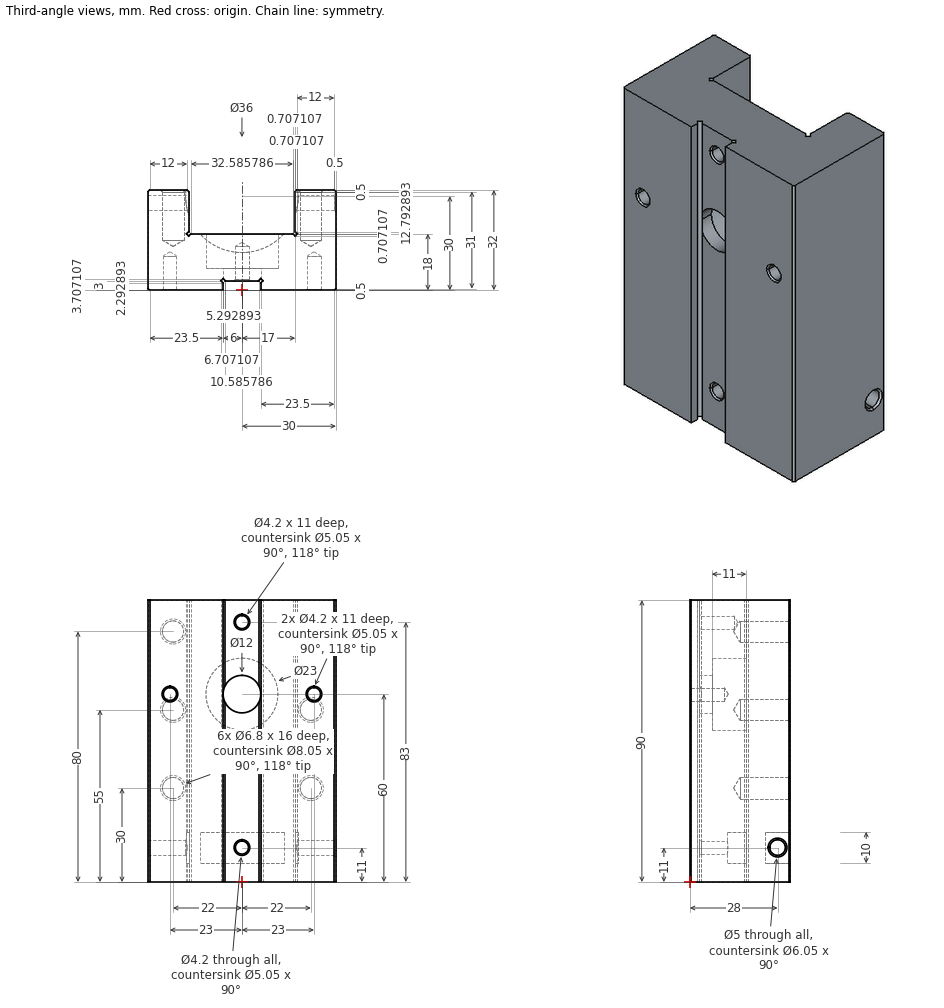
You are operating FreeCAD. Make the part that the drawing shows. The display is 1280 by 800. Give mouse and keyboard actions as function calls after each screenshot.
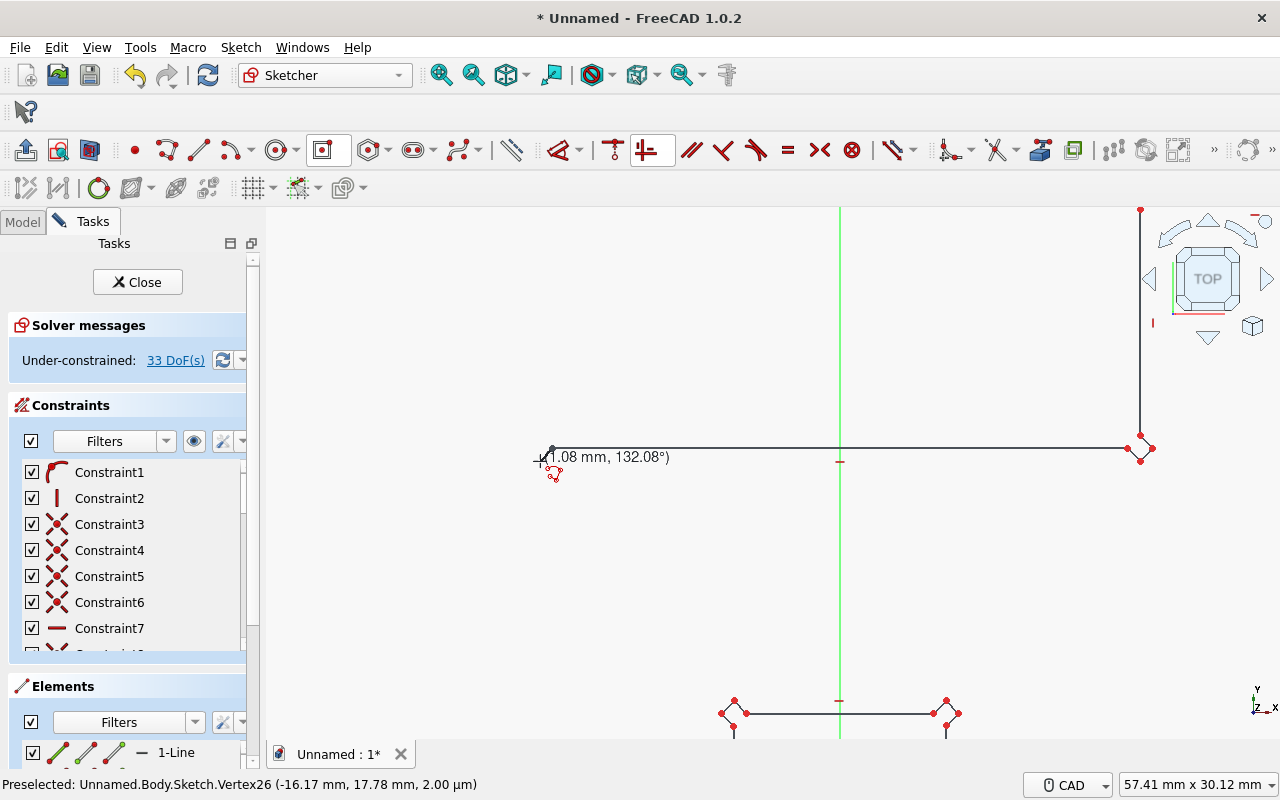
click(540, 460)
click(527, 448)
click(540, 435)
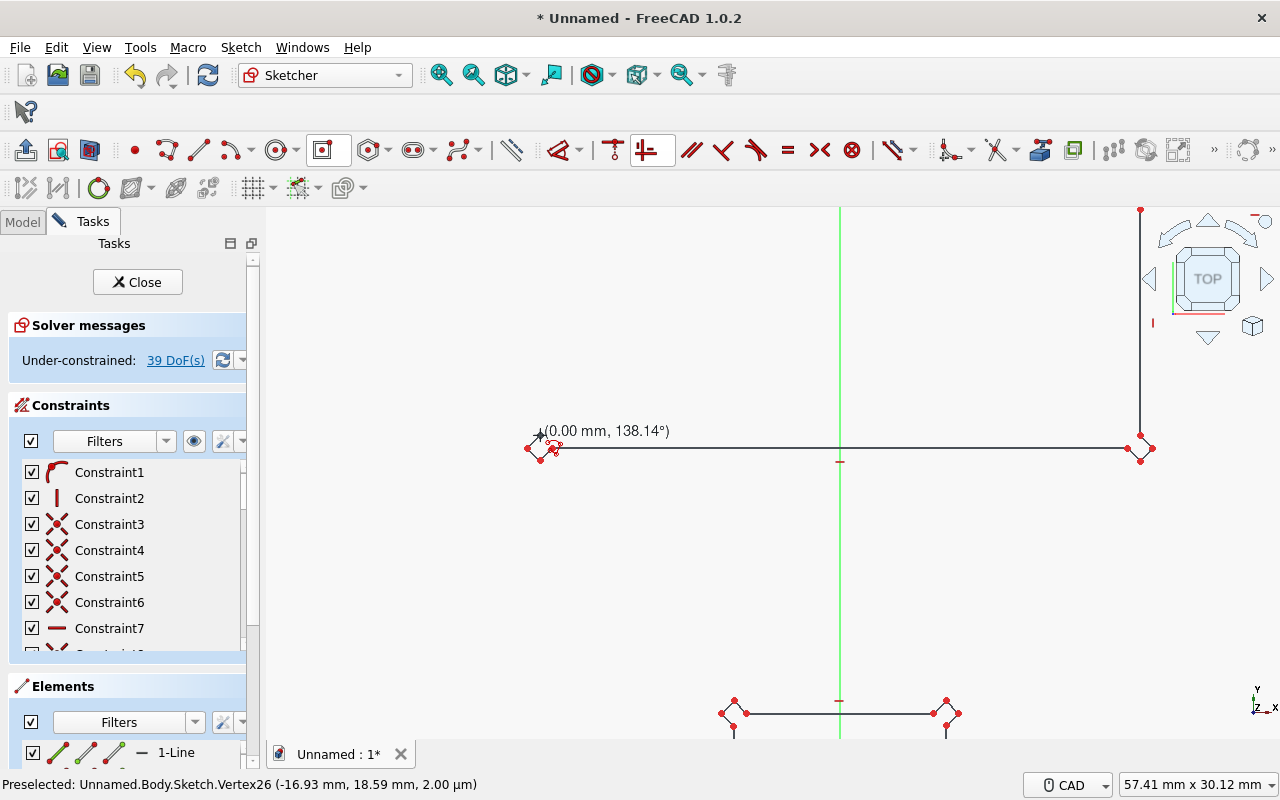
scroll(540, 461, down, 3)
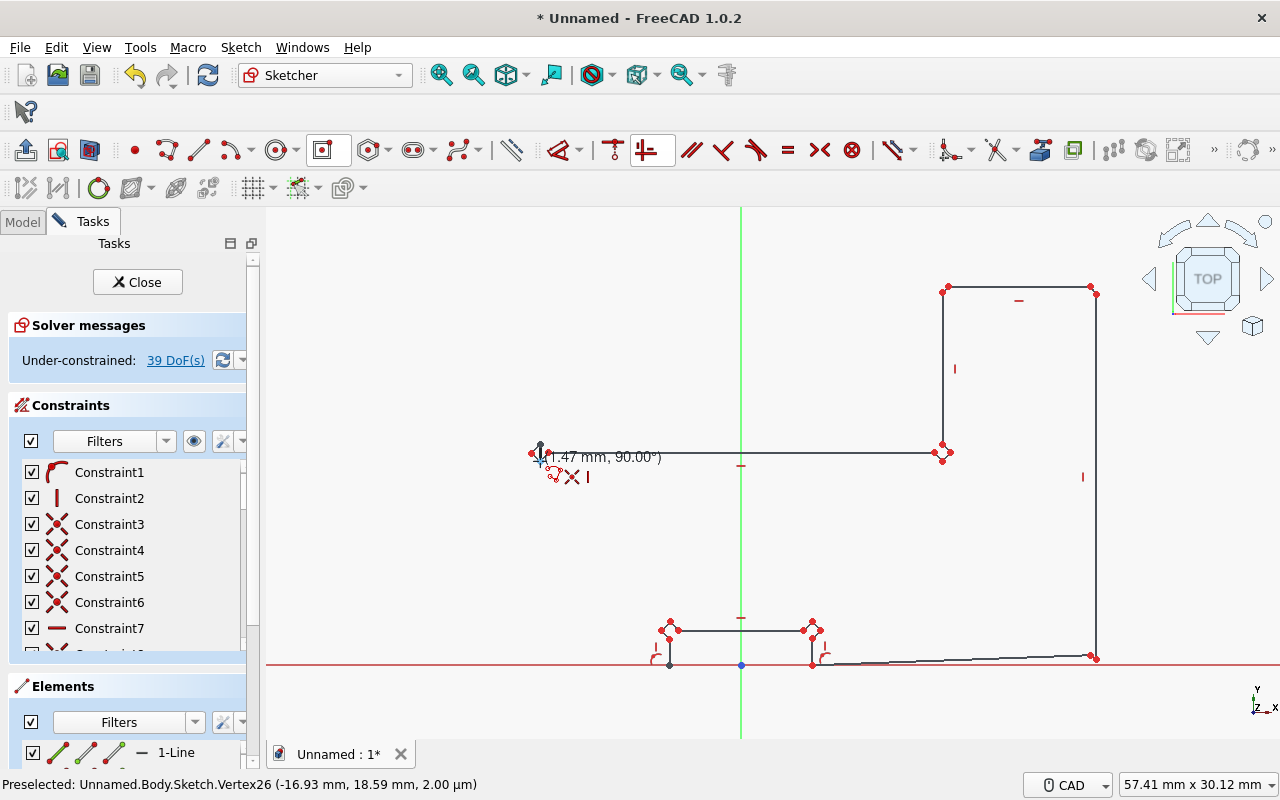
click(540, 323)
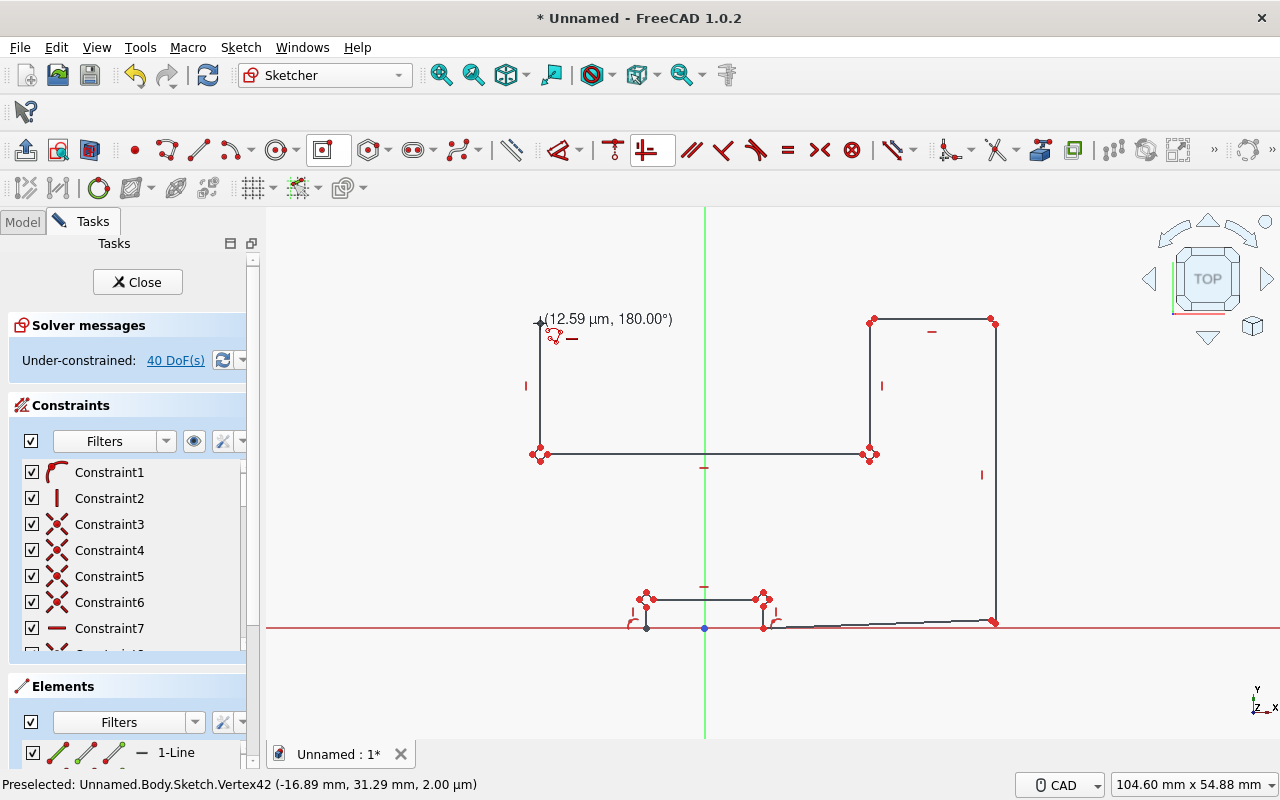
scroll(535, 318, up, 5)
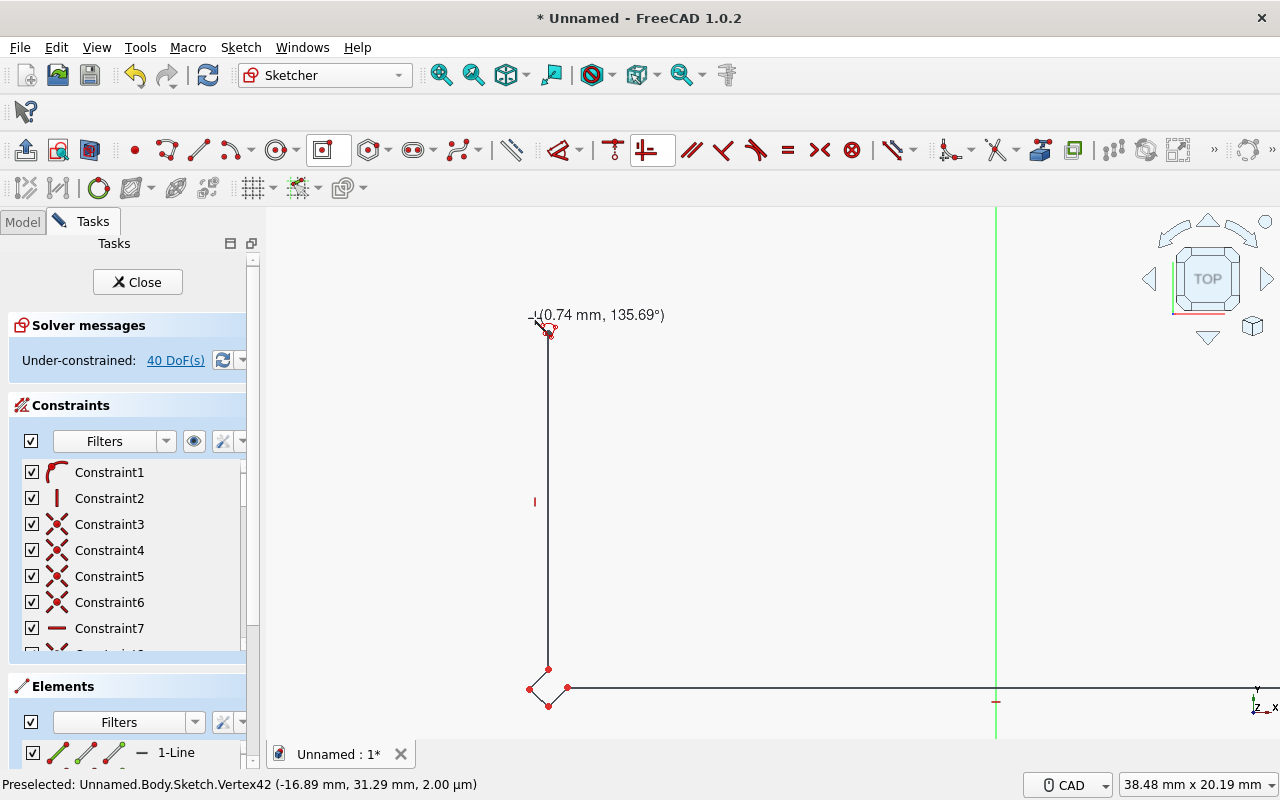
click(535, 318)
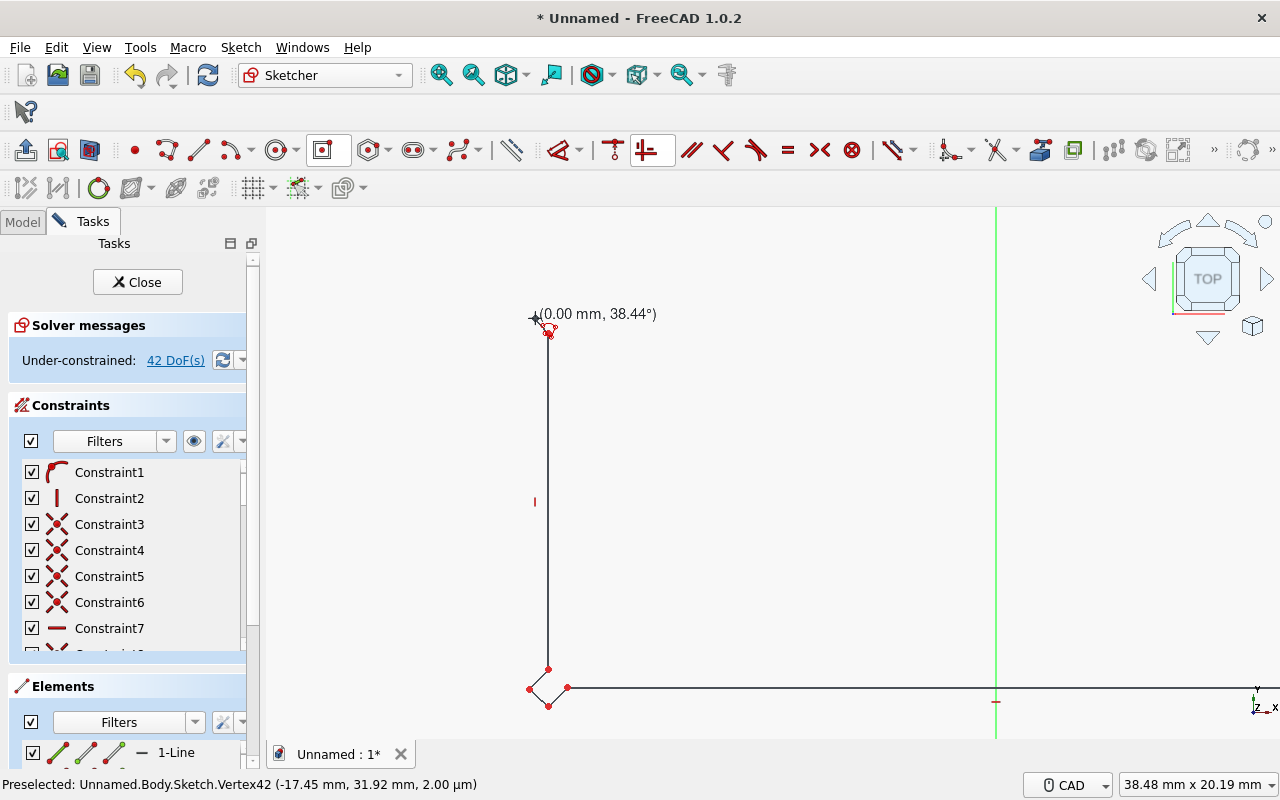
scroll(535, 318, down, 5)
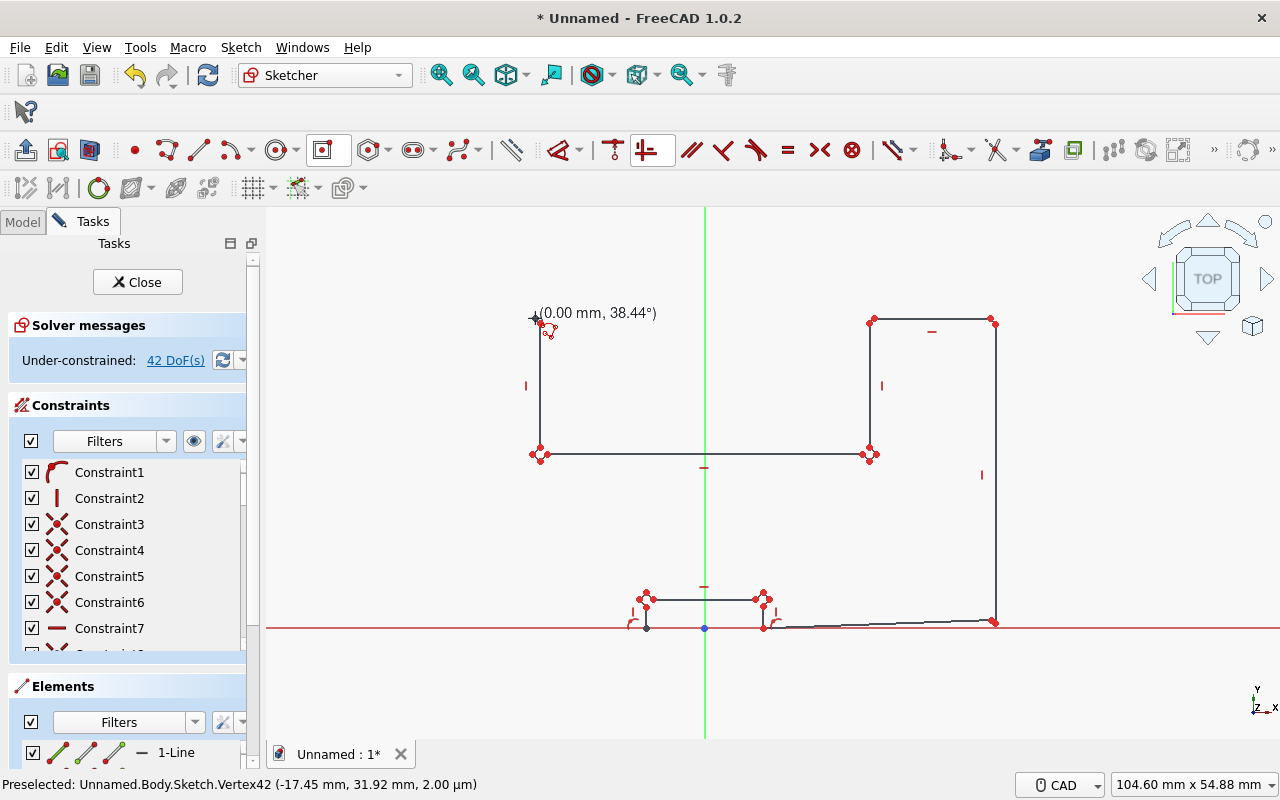
click(419, 318)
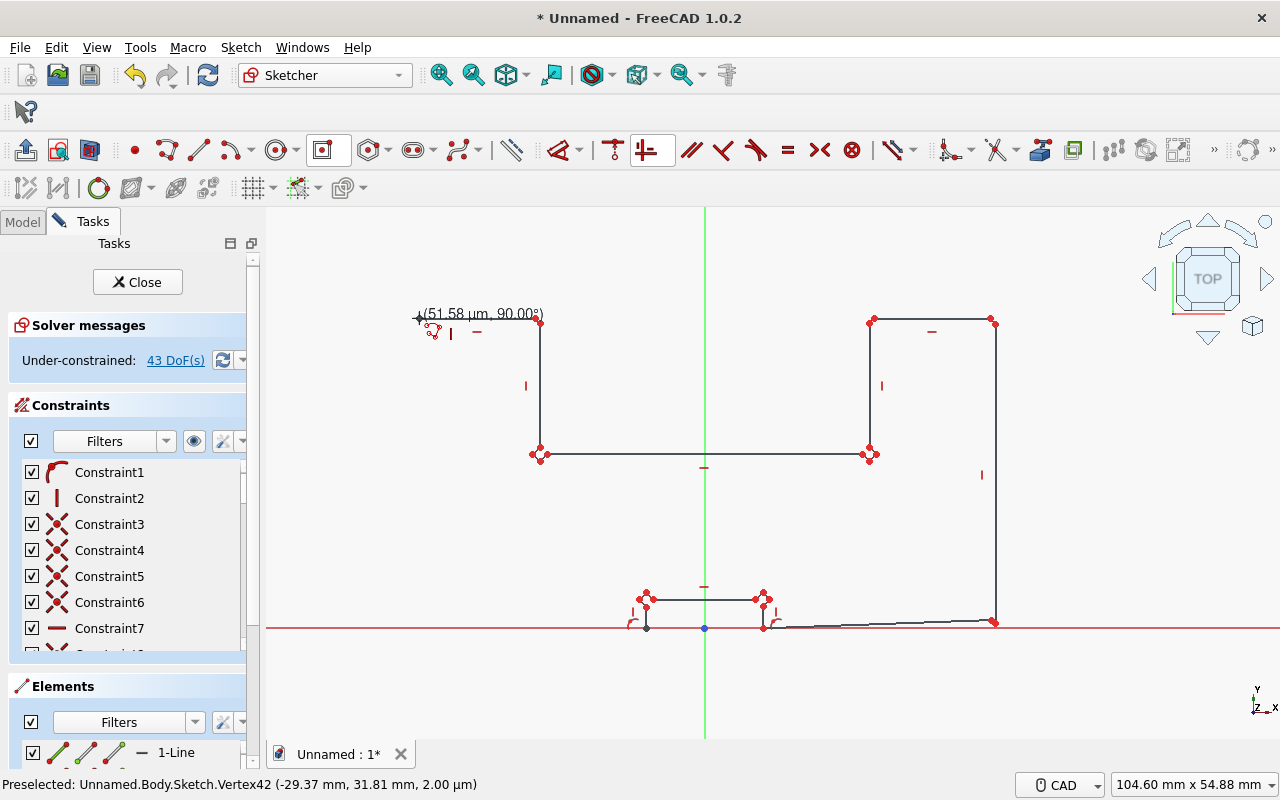
scroll(414, 323, up, 5)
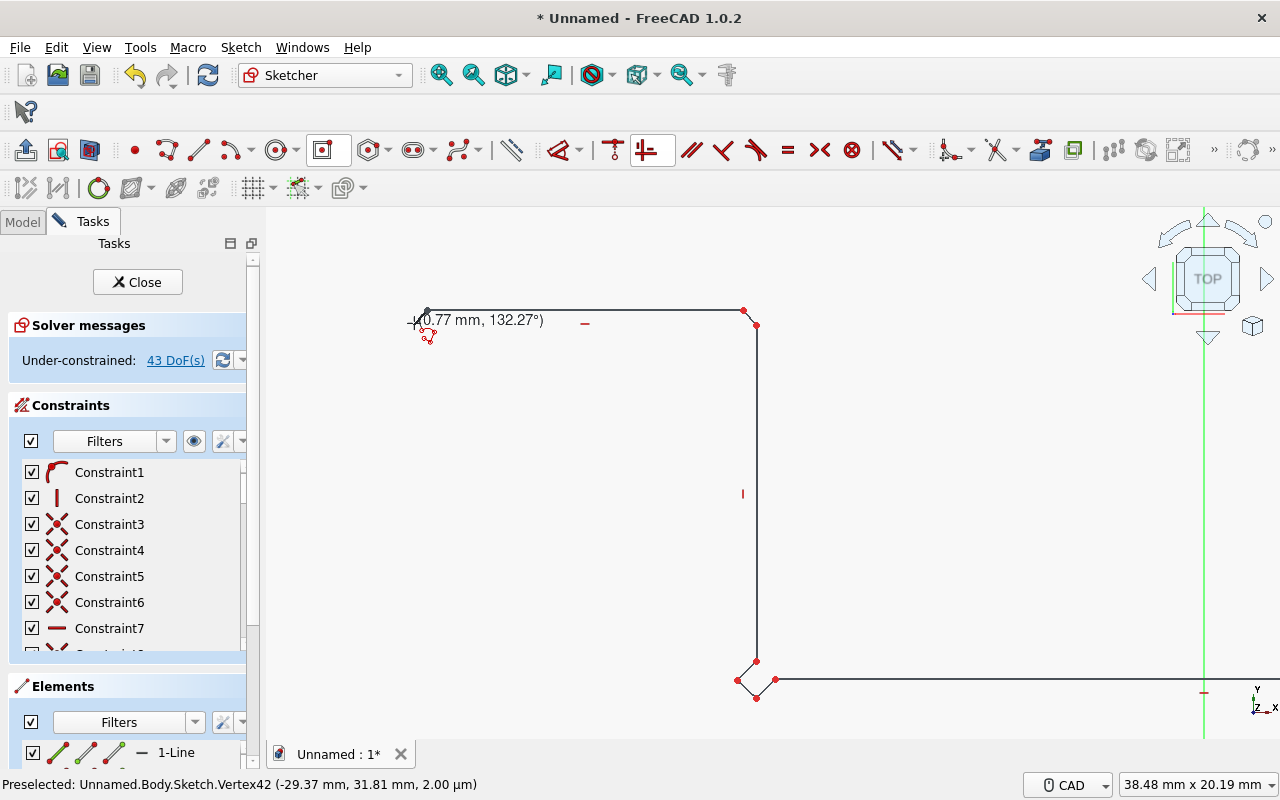
click(414, 323)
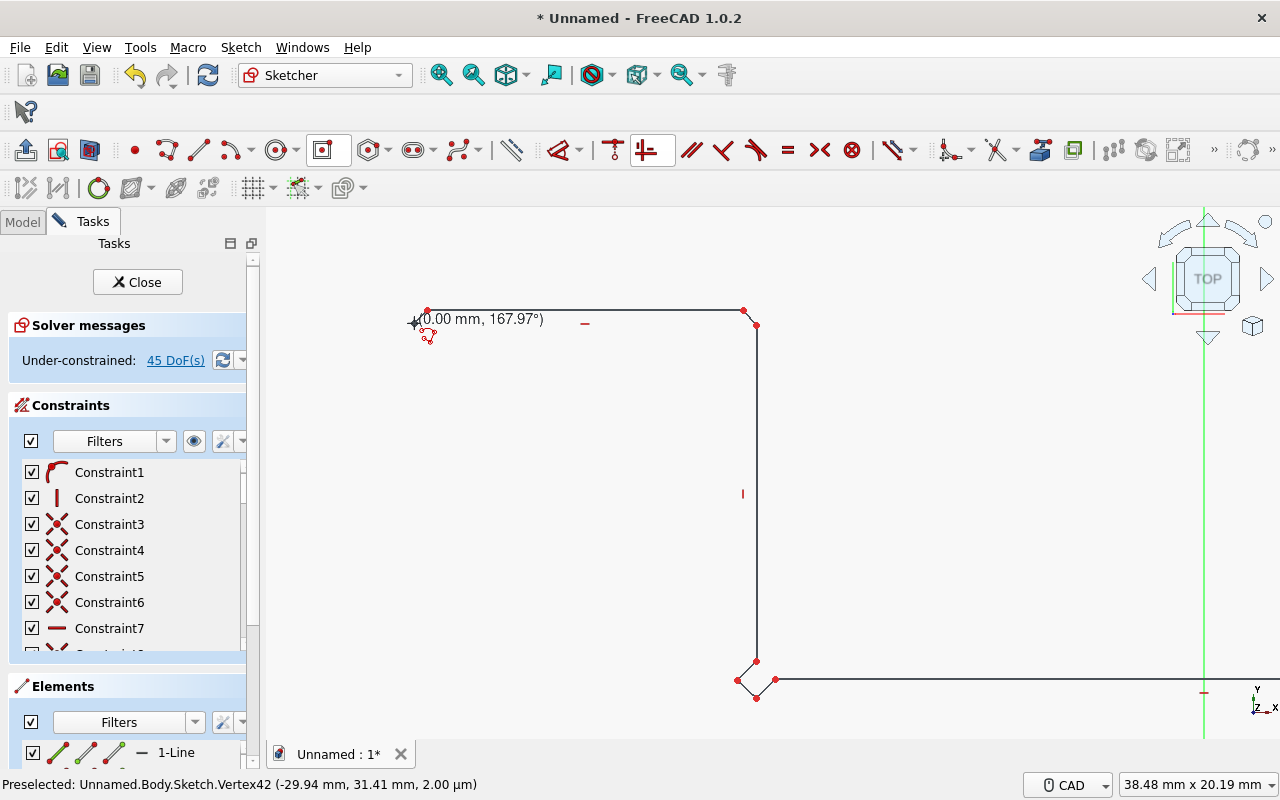
scroll(414, 323, down, 5)